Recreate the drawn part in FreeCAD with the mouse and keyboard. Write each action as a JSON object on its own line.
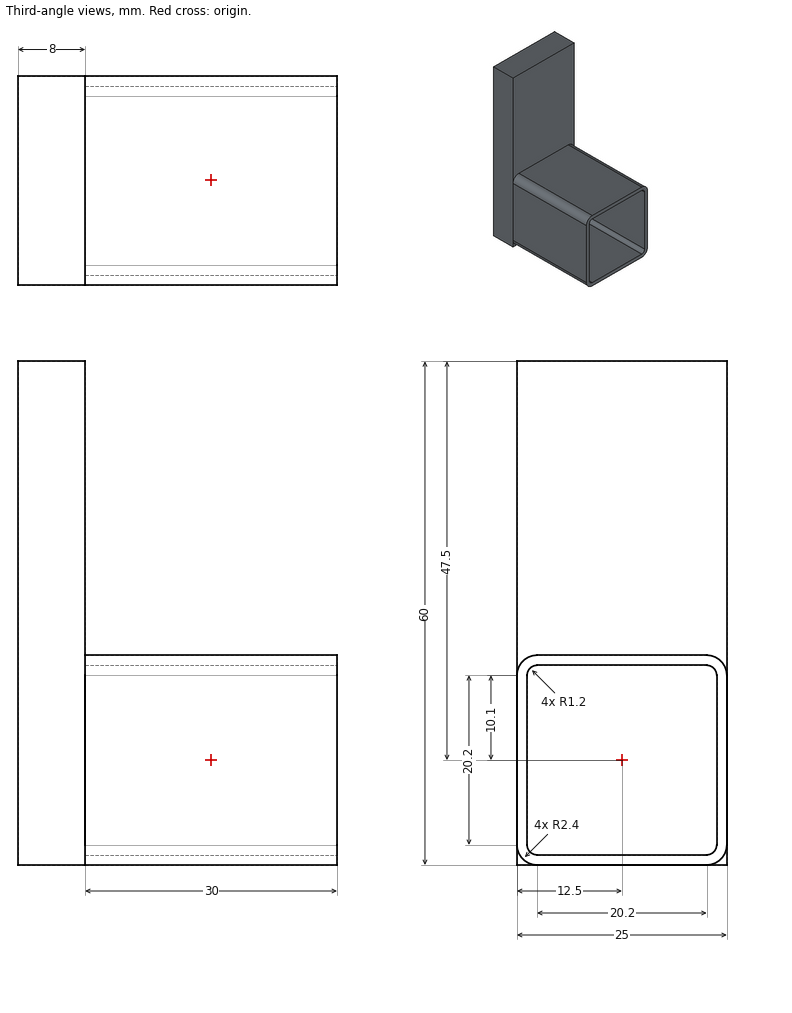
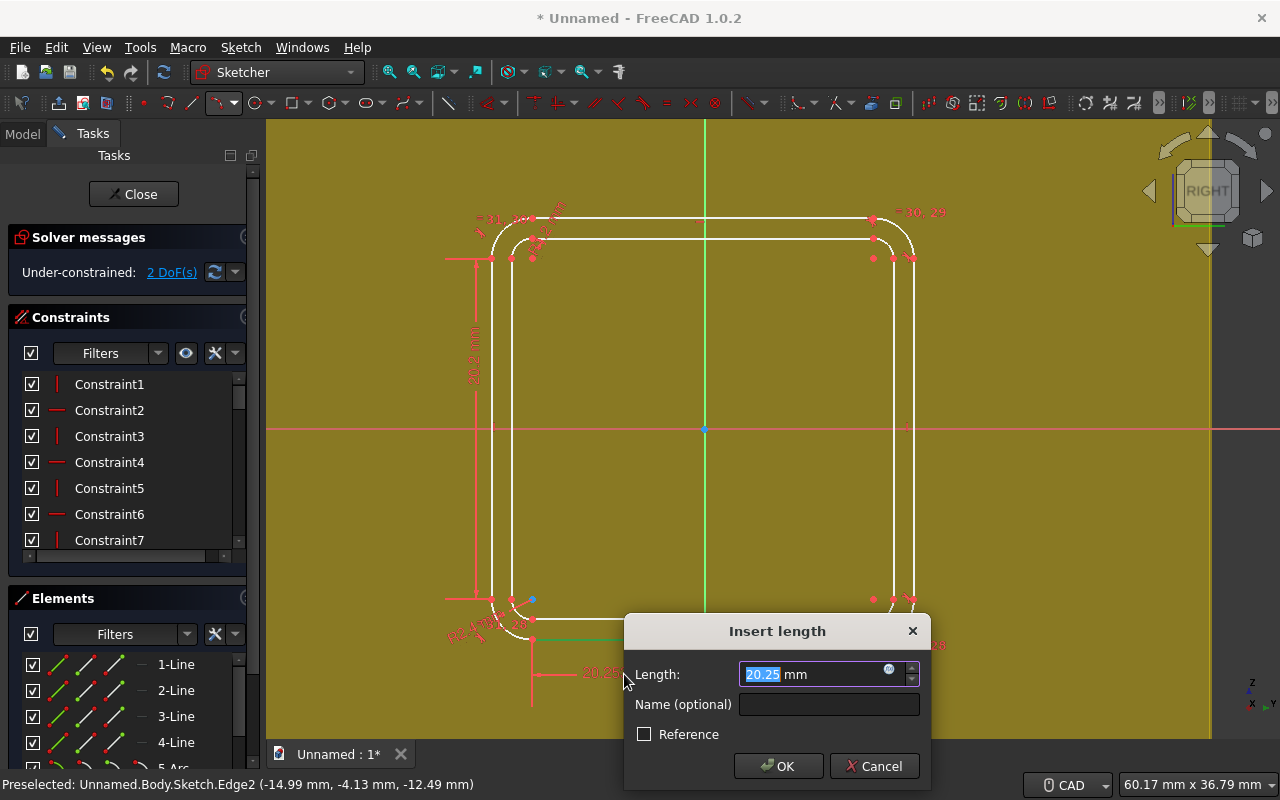
{"action": "type", "text": "20.2"}
{"action": "key", "text": "Return"}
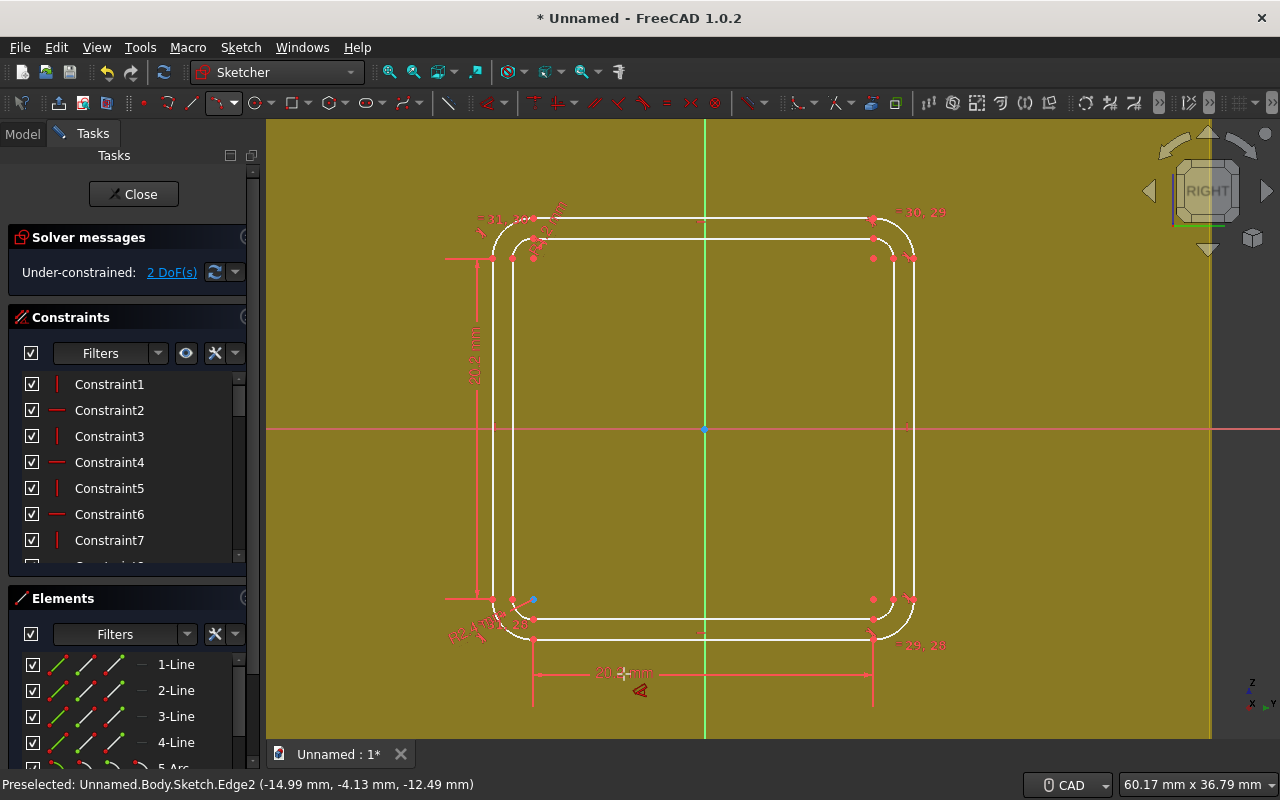
{"action": "left_click", "coordinate": [493, 259]}
{"action": "left_click", "coordinate": [599, 463]}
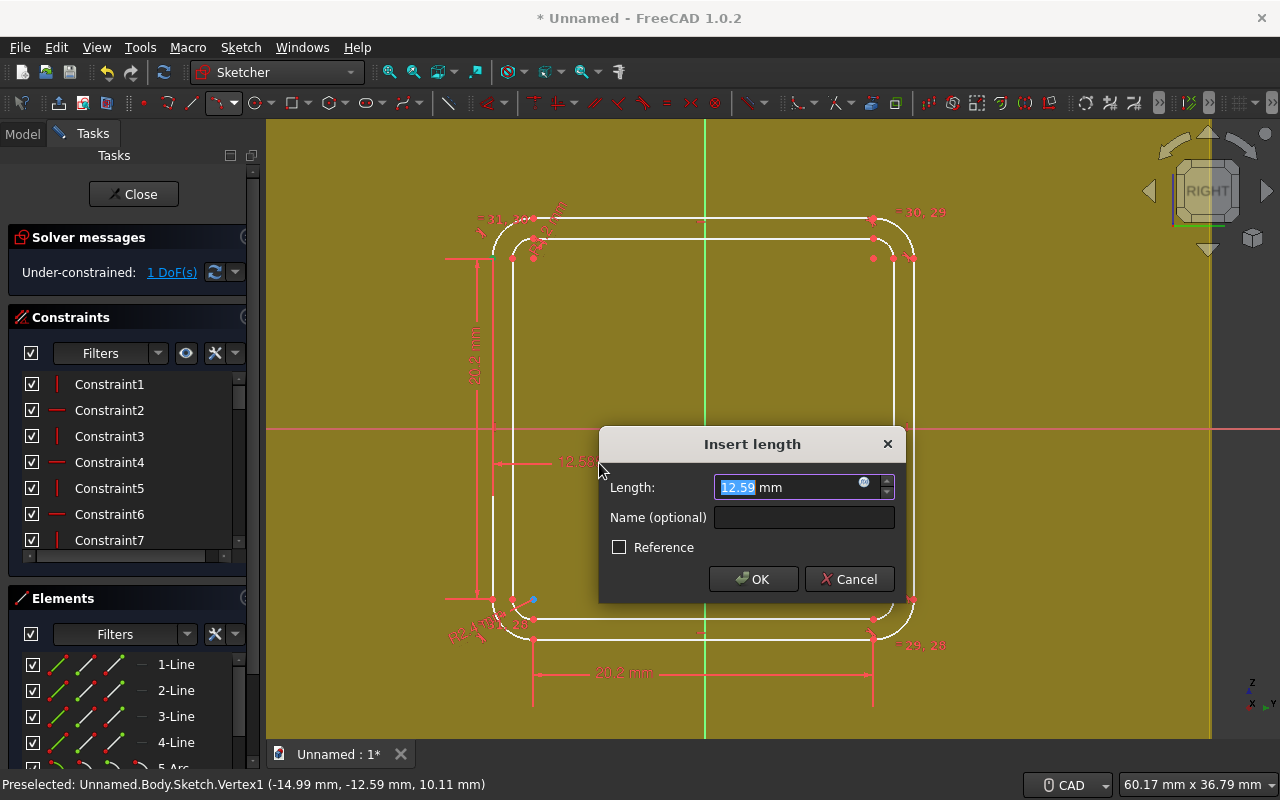
{"action": "type", "text": "12.5"}
{"action": "key", "text": "Return"}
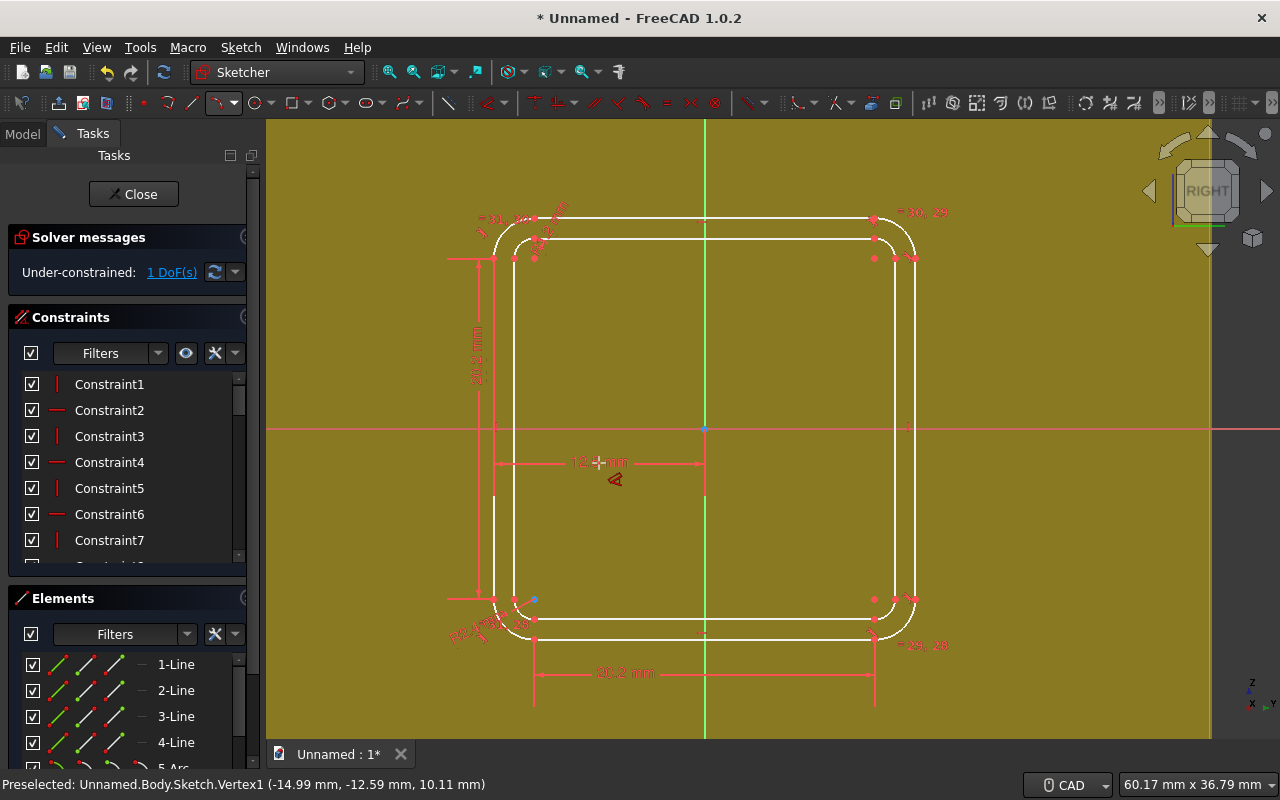
{"action": "left_click", "coordinate": [494, 259]}
{"action": "left_click", "coordinate": [460, 305]}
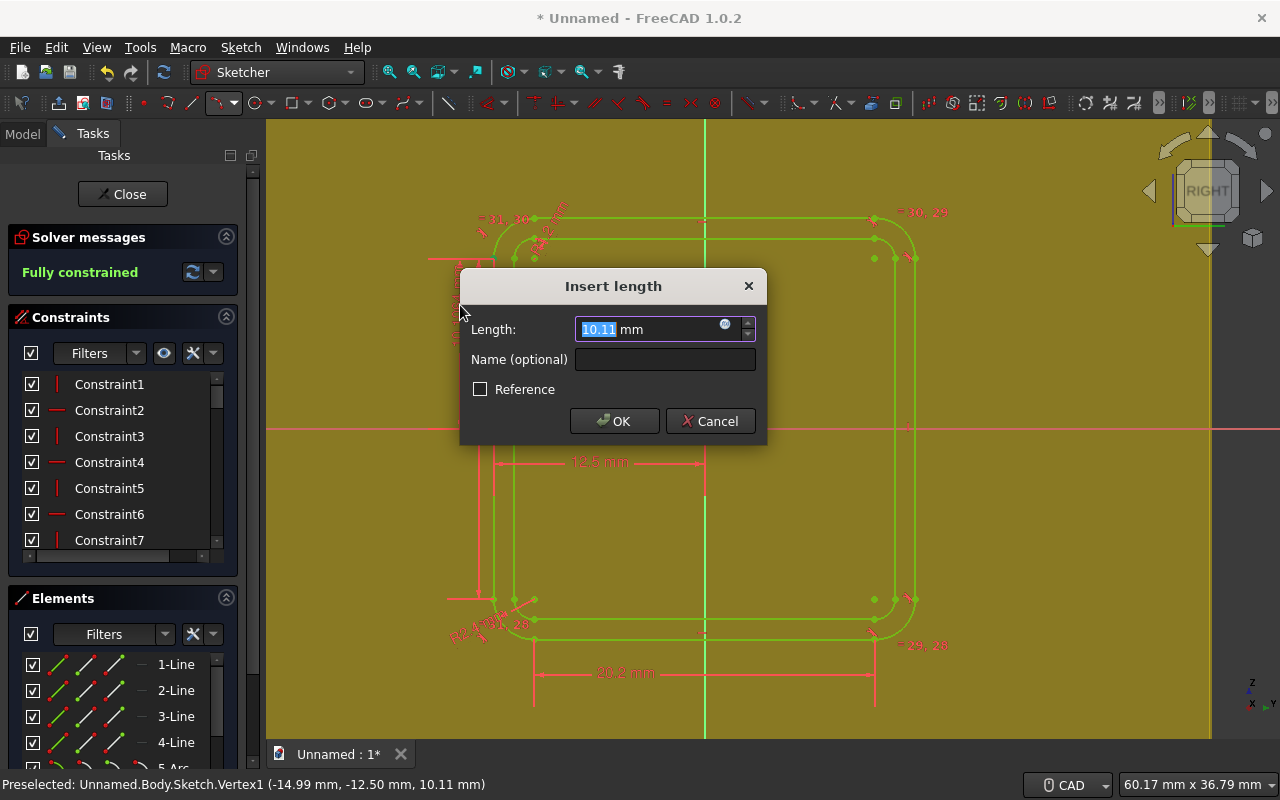
{"action": "type", "text": "10.1"}
{"action": "key", "text": "Return"}
{"action": "key", "text": "Escape"}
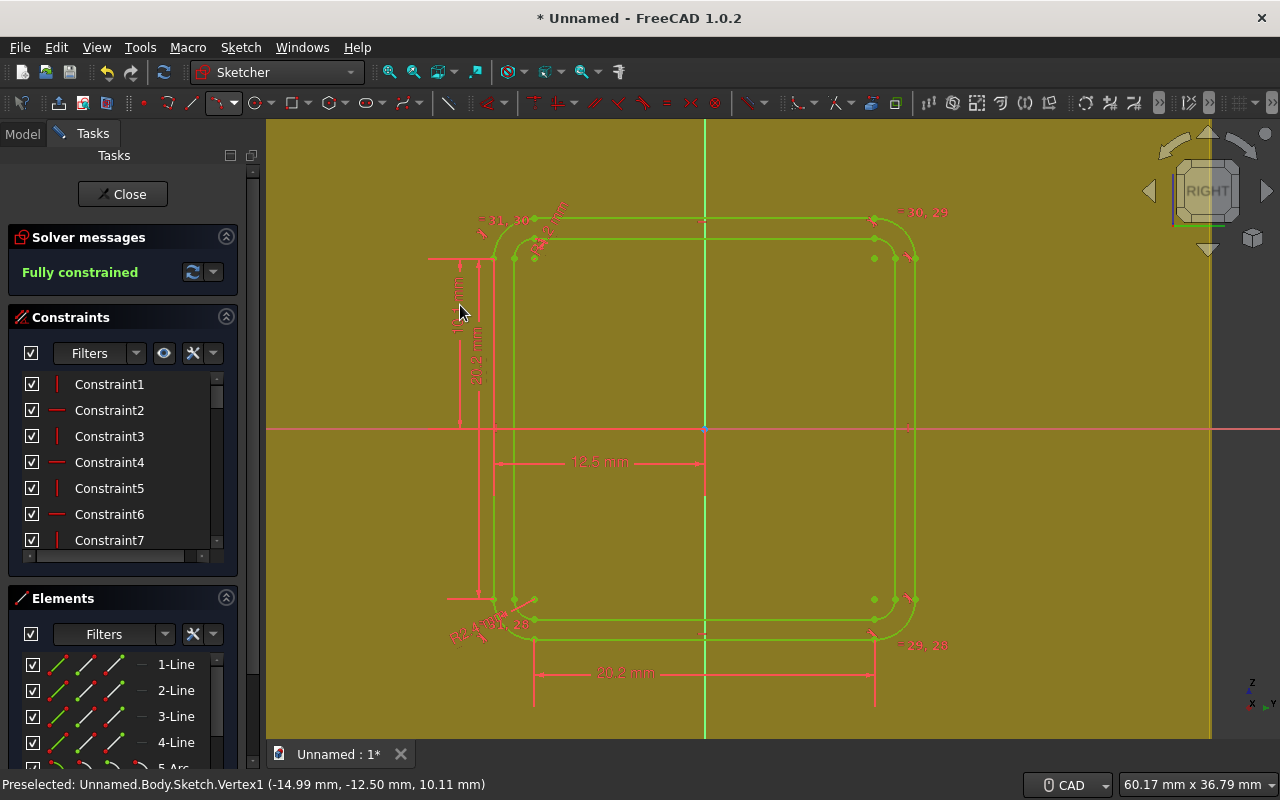
{"action": "left_click", "coordinate": [123, 194]}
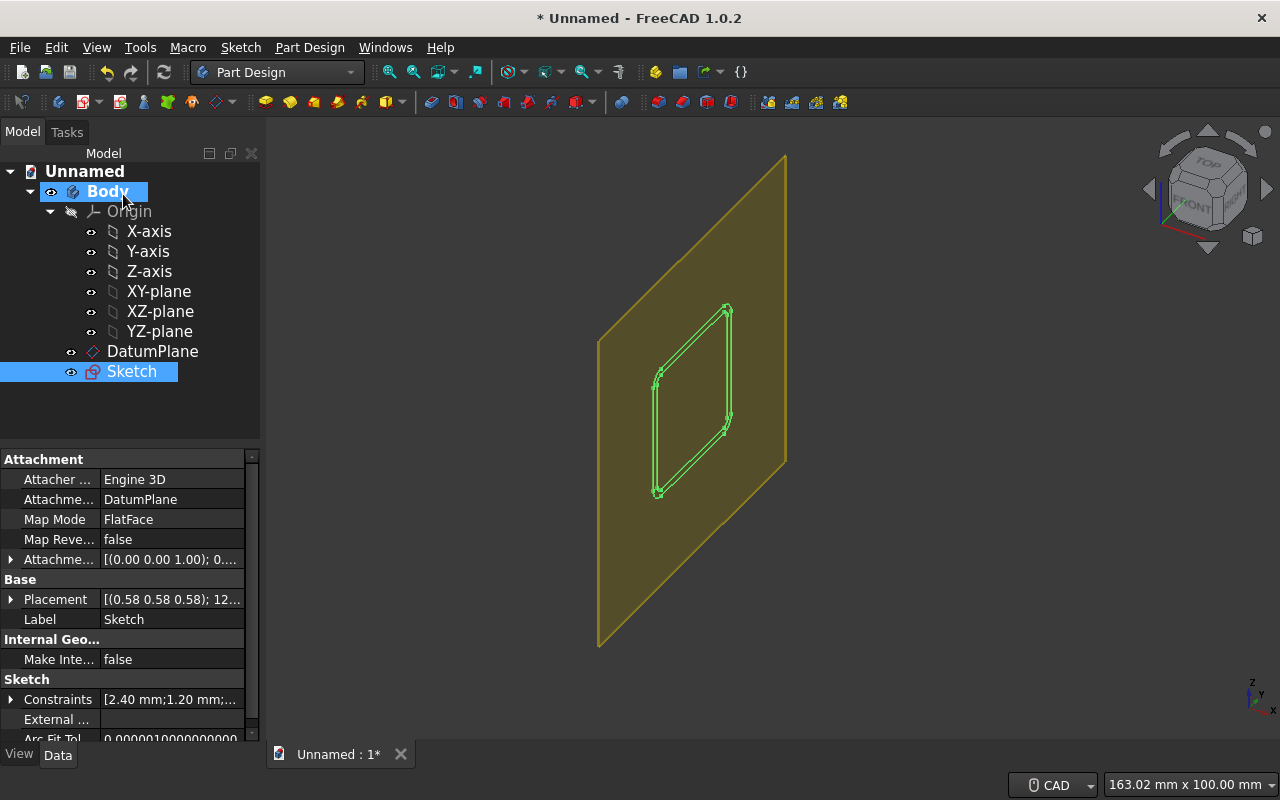
{"action": "left_click", "coordinate": [266, 102]}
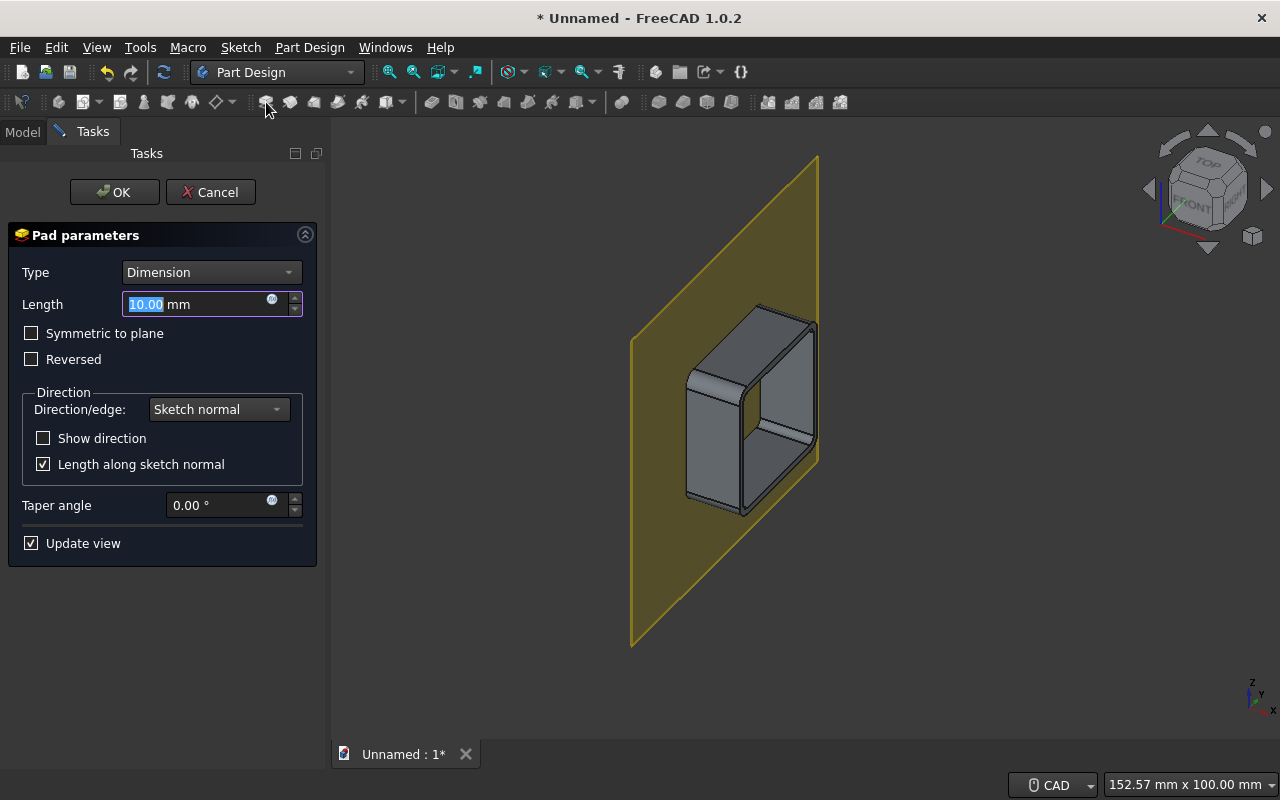
{"action": "type", "text": "30"}
{"action": "key", "text": "Tab"}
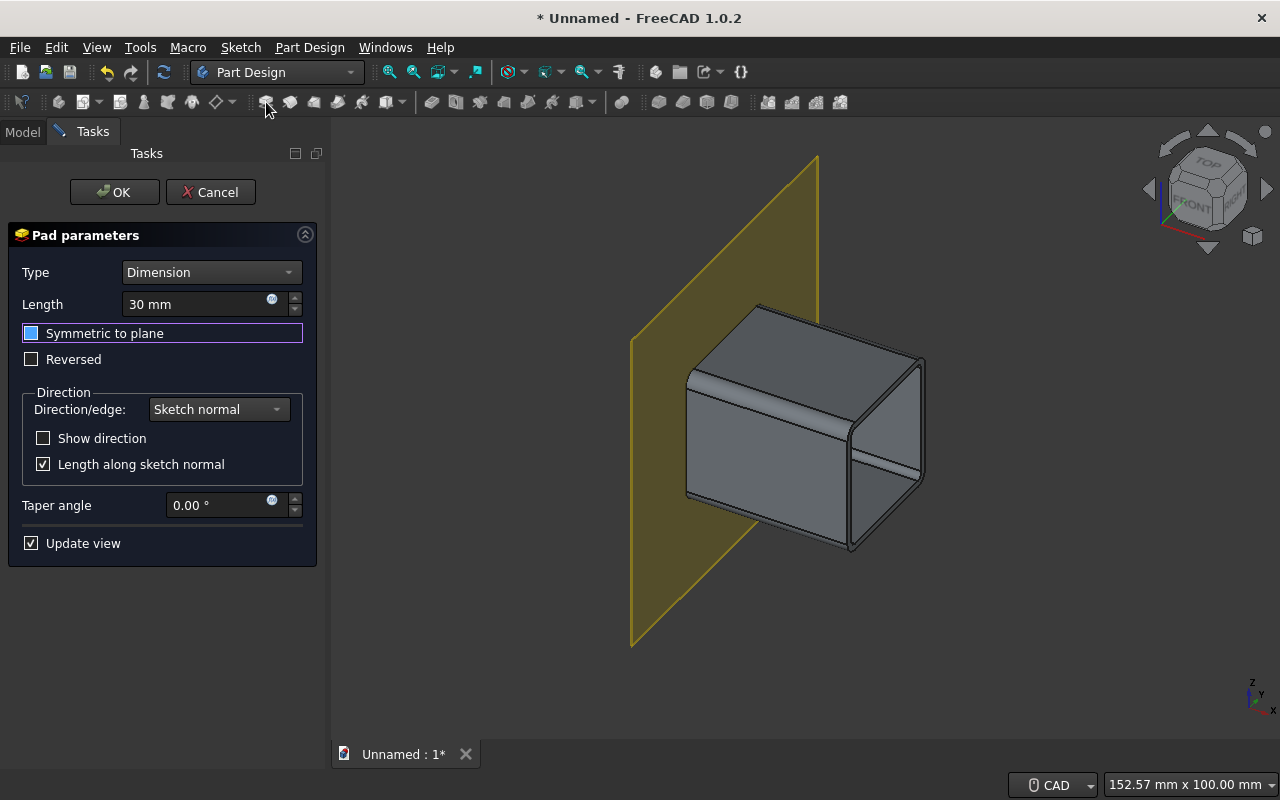
{"action": "left_click", "coordinate": [115, 192]}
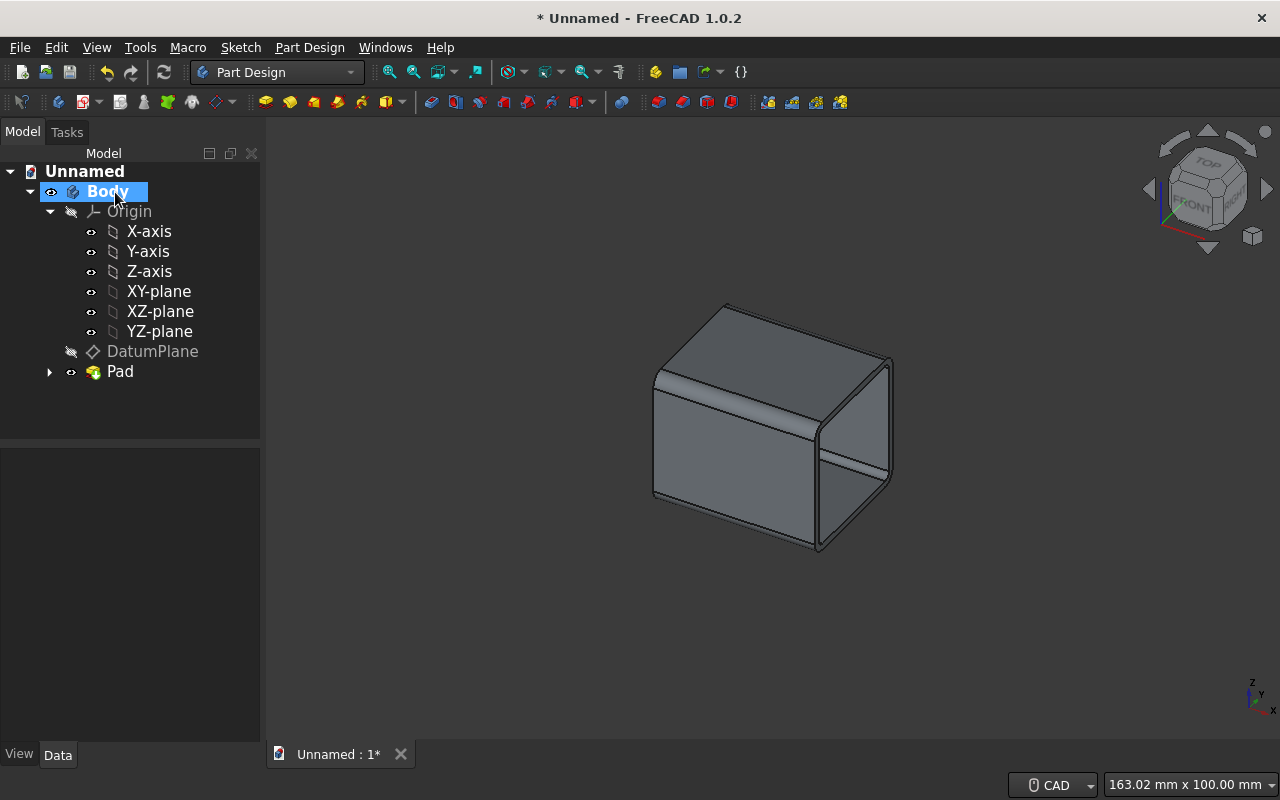
{"action": "key", "text": "v f"}